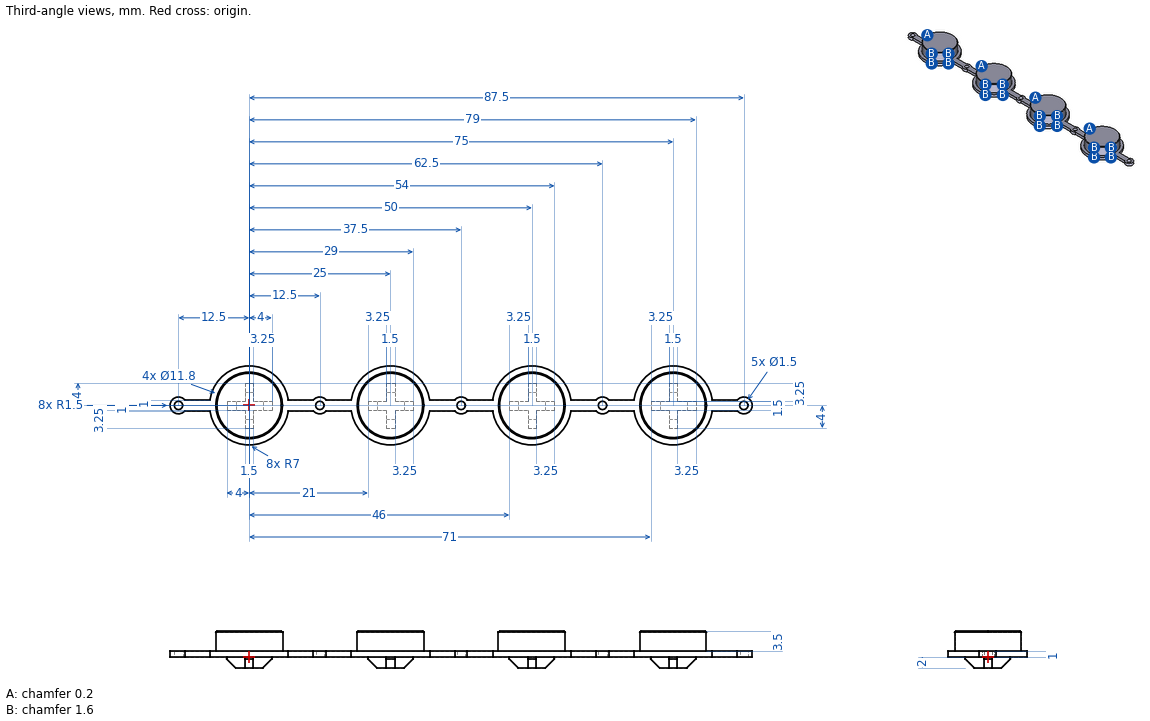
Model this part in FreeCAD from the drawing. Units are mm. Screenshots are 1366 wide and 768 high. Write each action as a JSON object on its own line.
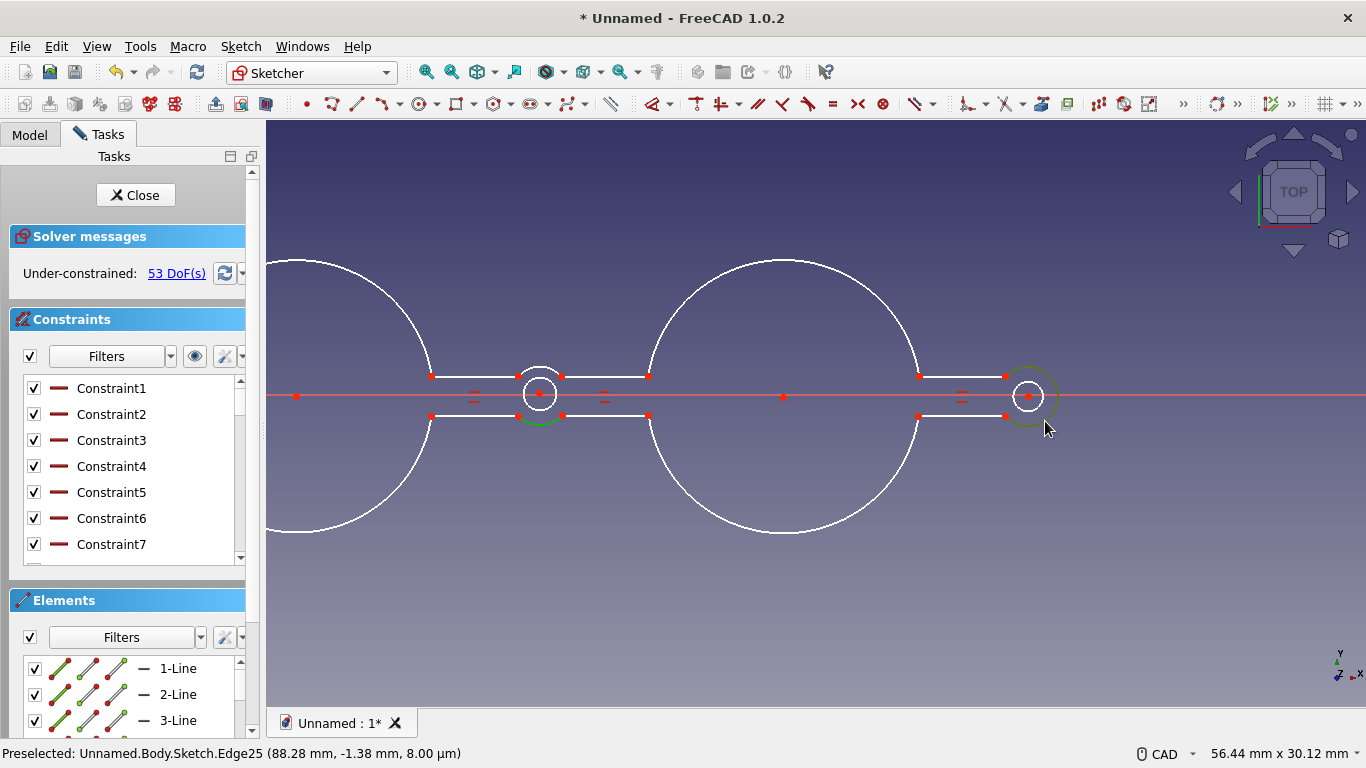
{"action": "scroll", "coordinate": [550, 368], "scroll_direction": "up", "scroll_amount": 2}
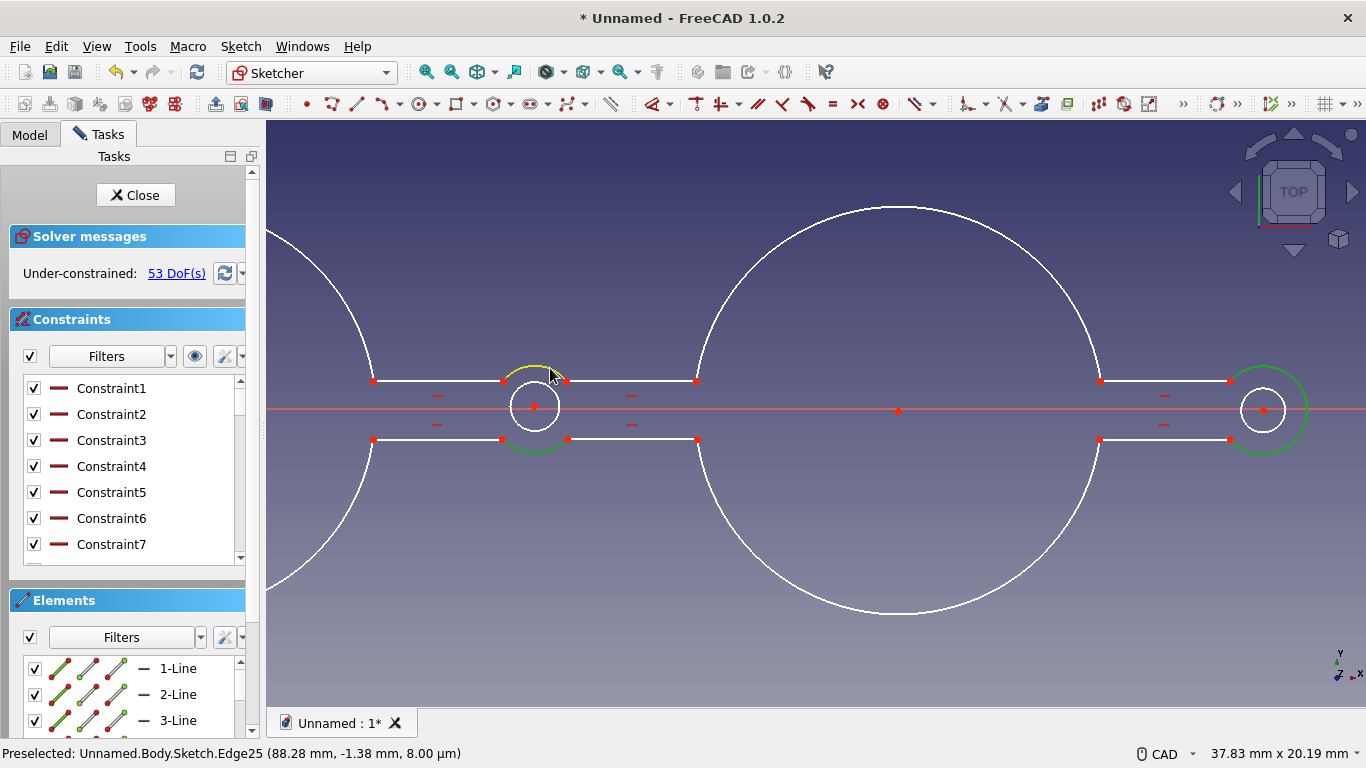
{"action": "left_click", "coordinate": [549, 368]}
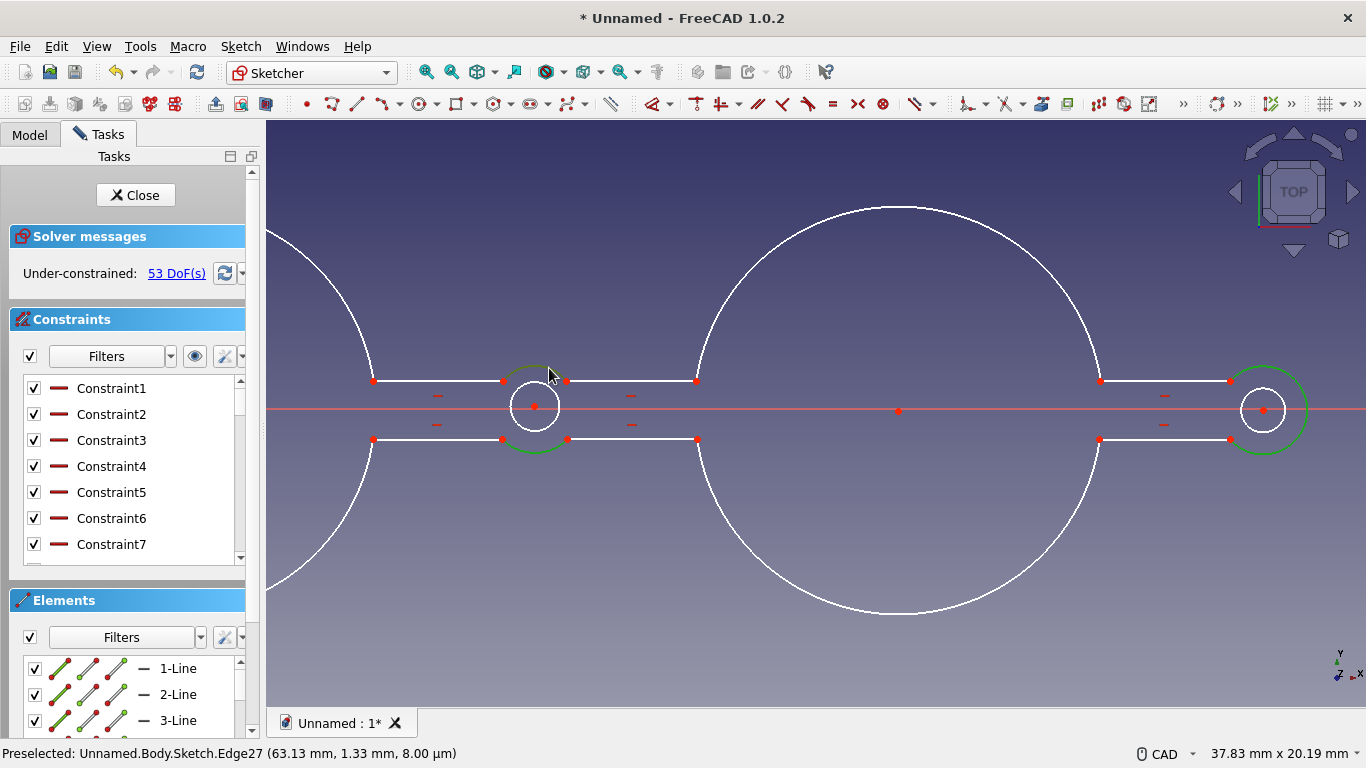
{"action": "scroll", "coordinate": [985, 415], "scroll_direction": "down", "scroll_amount": 8}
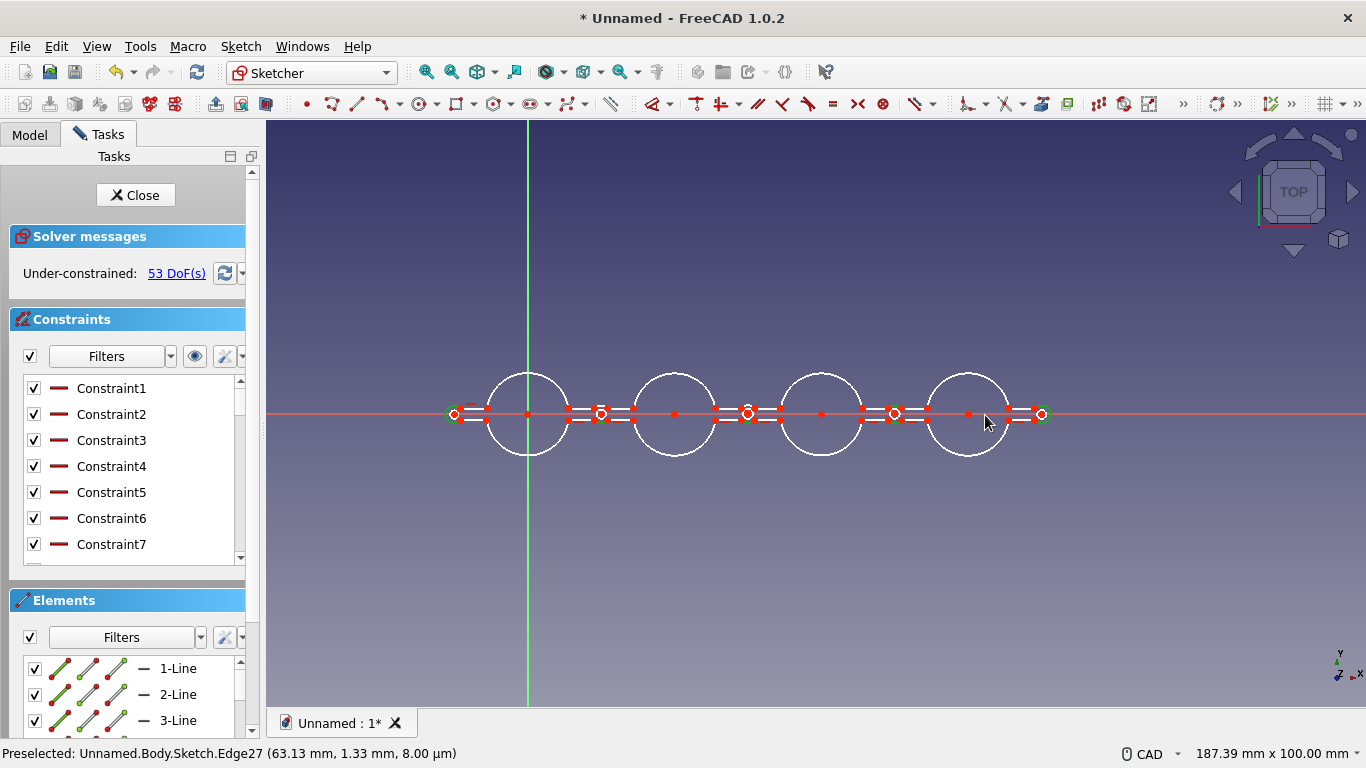
{"action": "scroll", "coordinate": [751, 406], "scroll_direction": "up", "scroll_amount": 7}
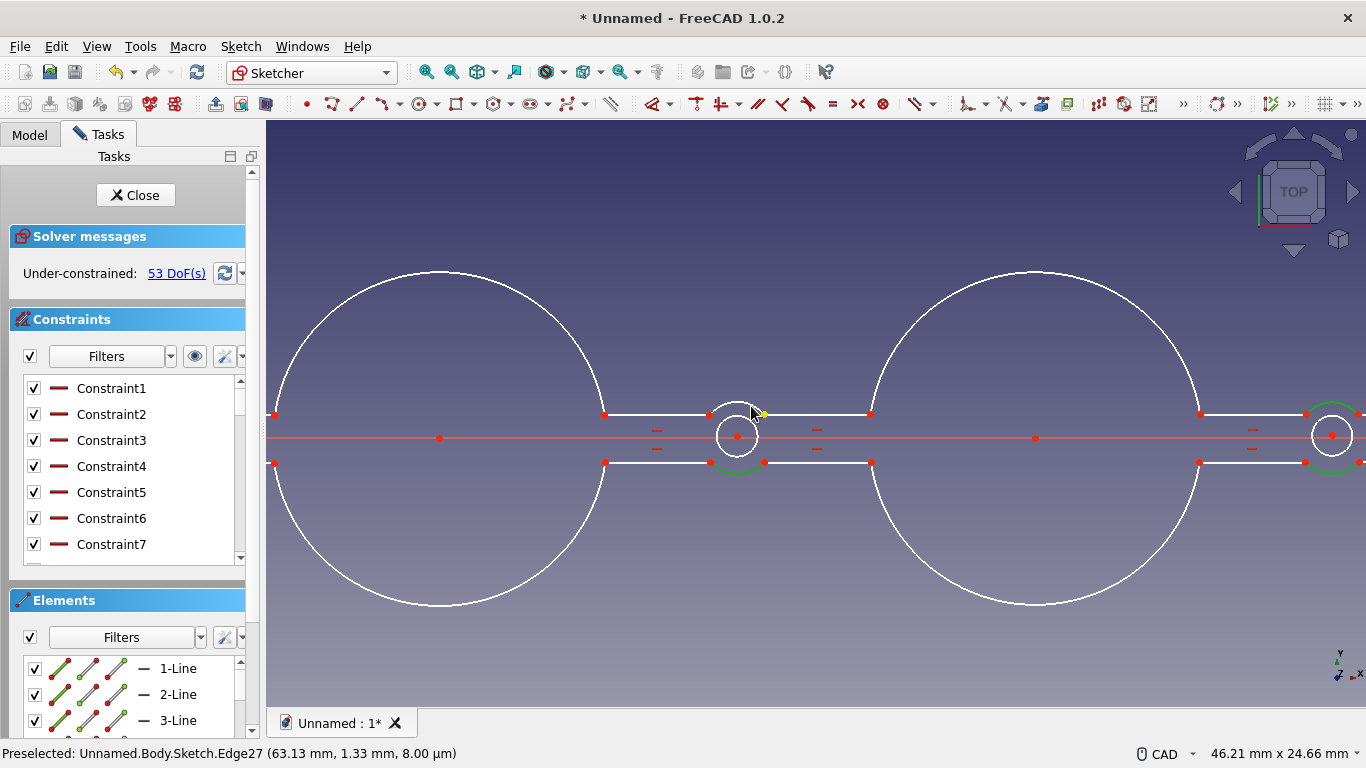
{"action": "left_click", "coordinate": [749, 404]}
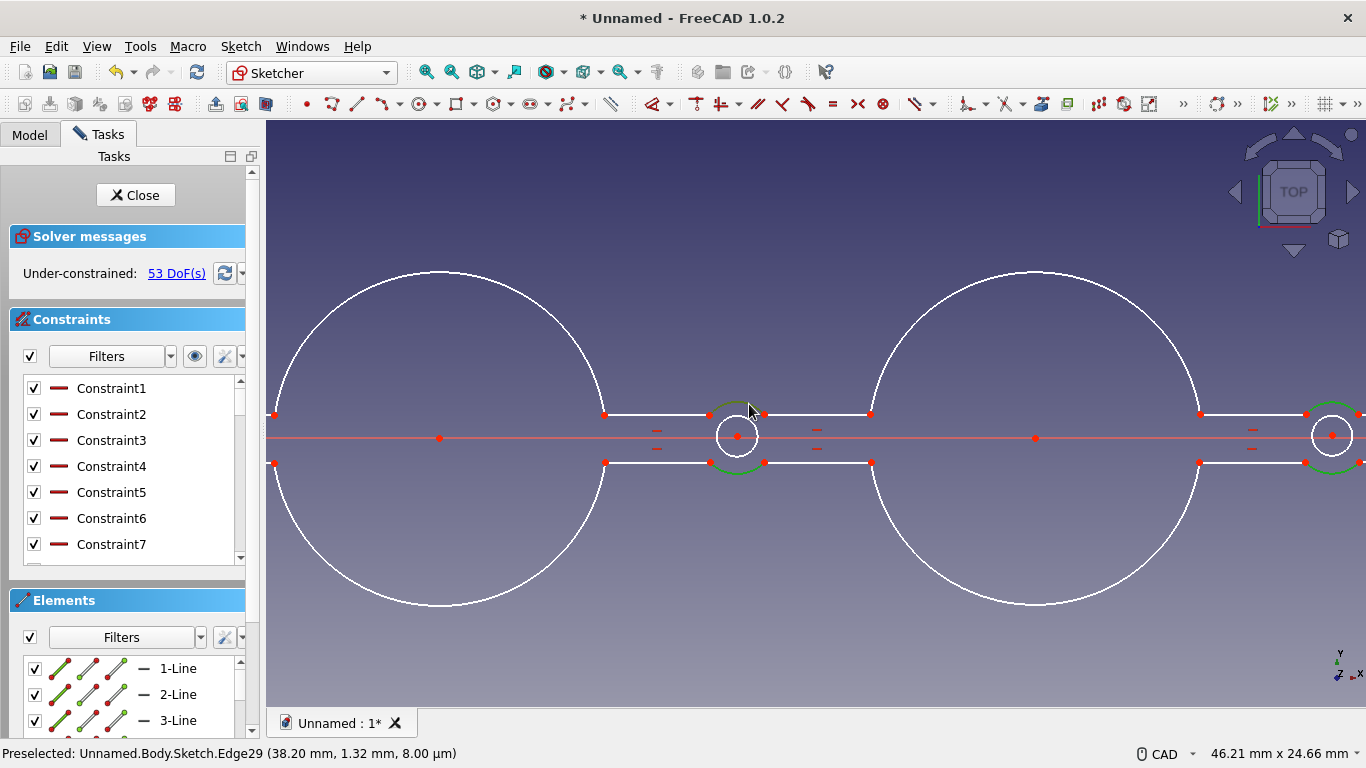
{"action": "scroll", "coordinate": [751, 406], "scroll_direction": "down", "scroll_amount": 7}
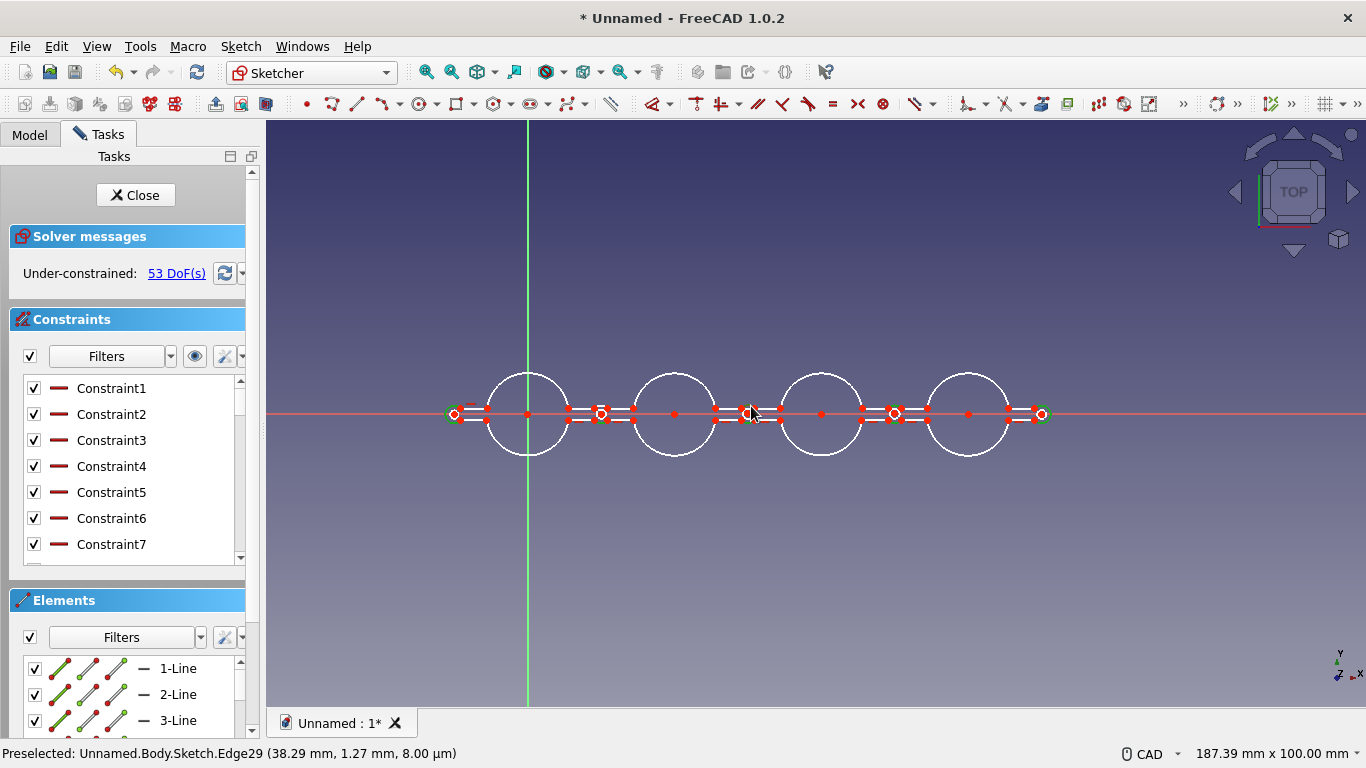
{"action": "scroll", "coordinate": [604, 406], "scroll_direction": "up", "scroll_amount": 7}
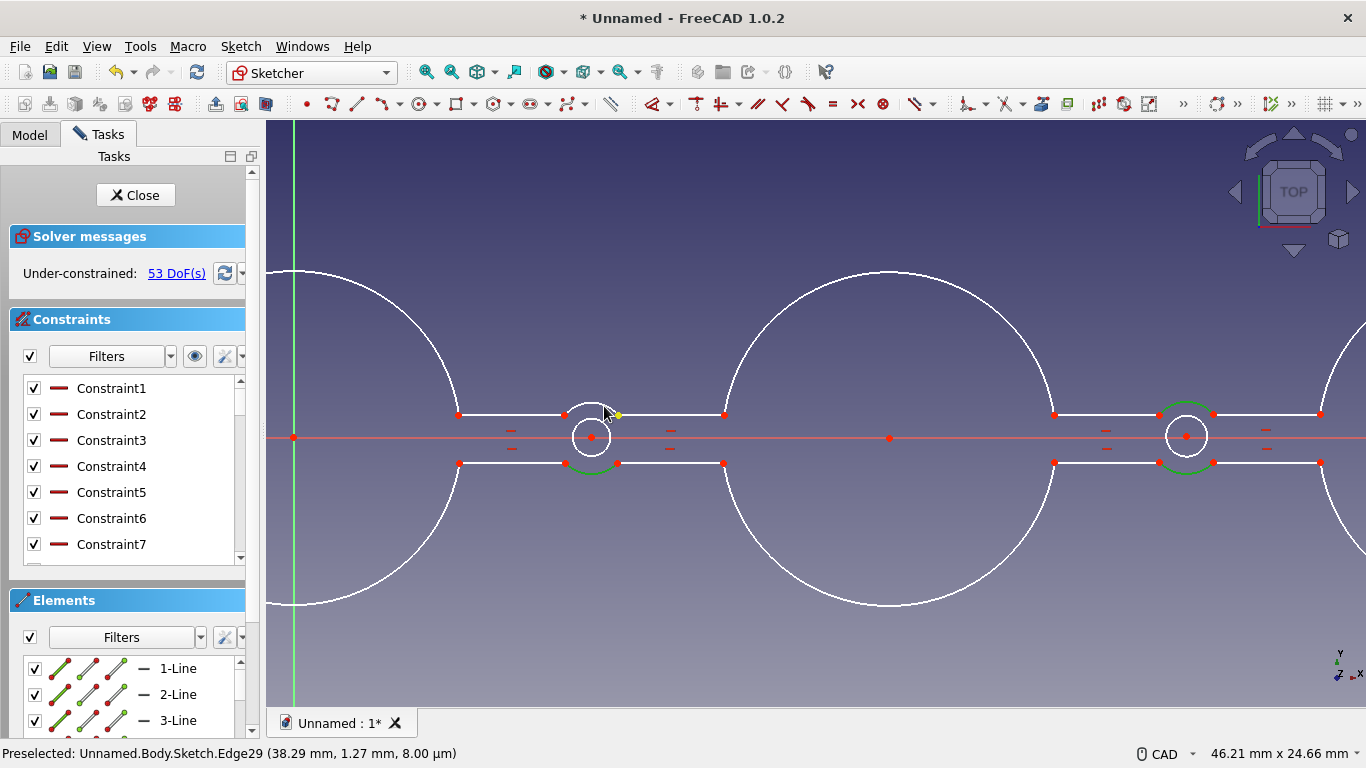
{"action": "left_click", "coordinate": [604, 405]}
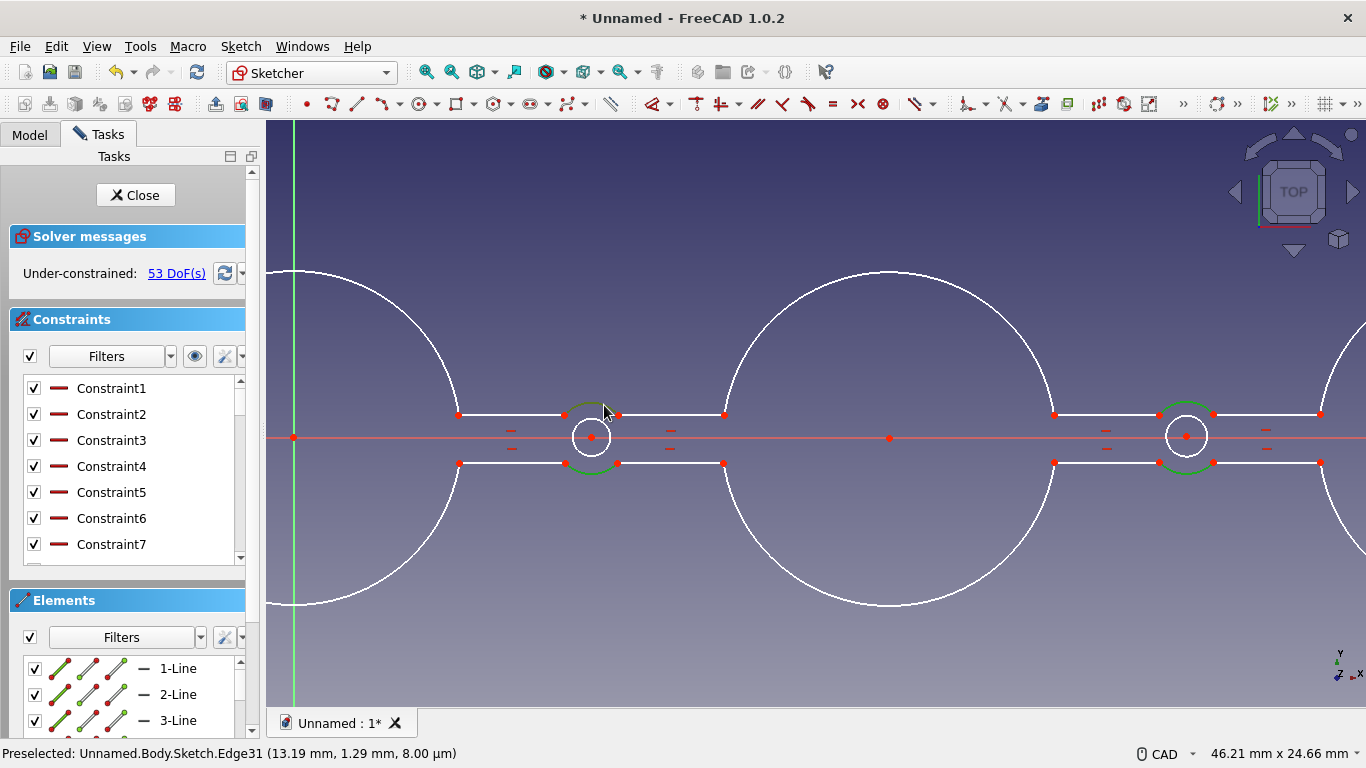
{"action": "key", "text": "e"}